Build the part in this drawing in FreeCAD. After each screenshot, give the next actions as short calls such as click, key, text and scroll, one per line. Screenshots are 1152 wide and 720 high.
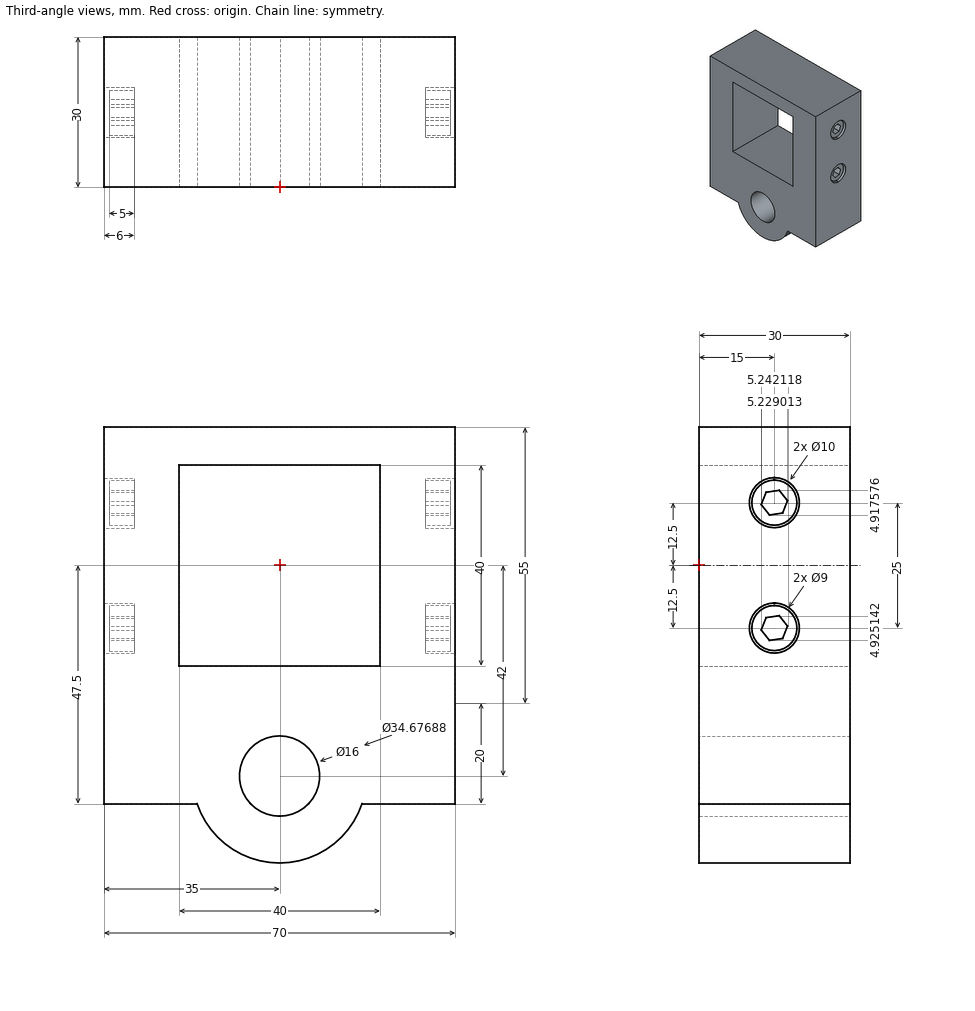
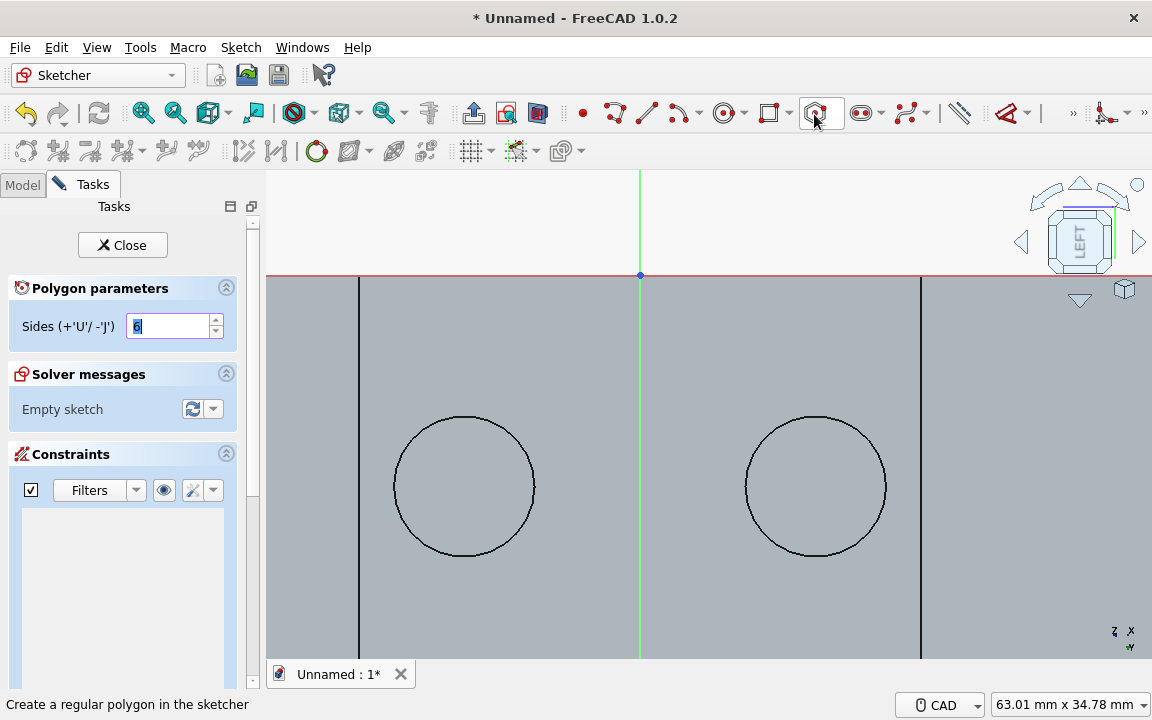
click(816, 487)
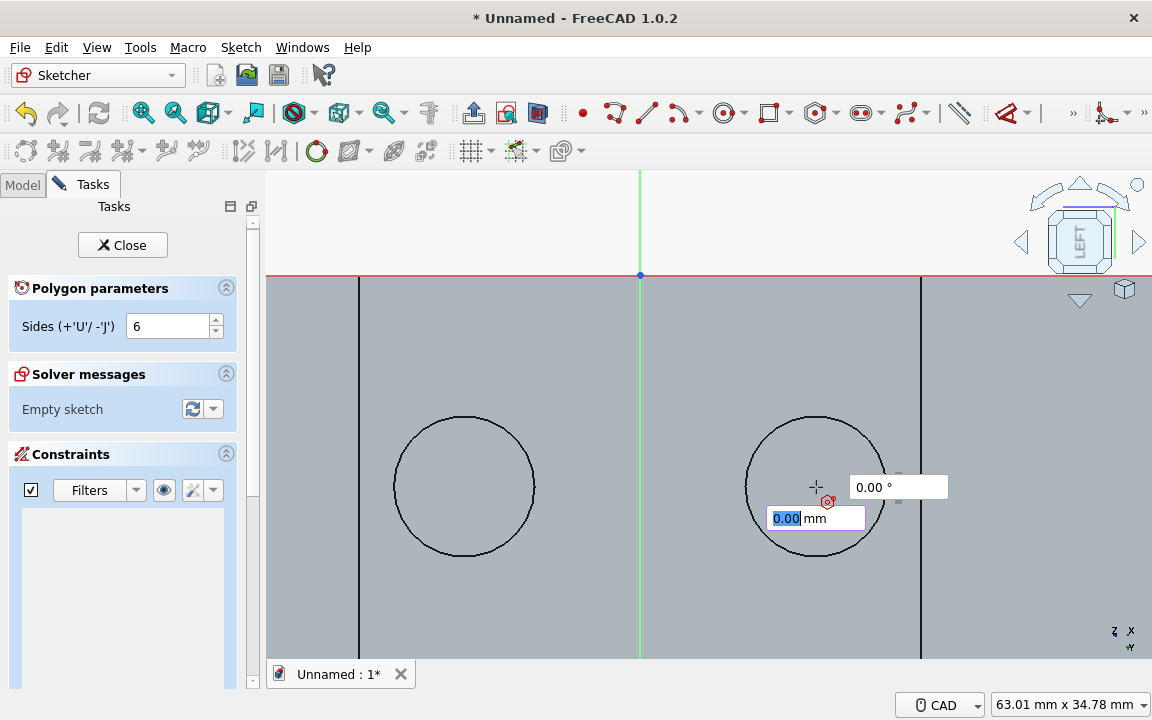
click(845, 510)
right_click(845, 510)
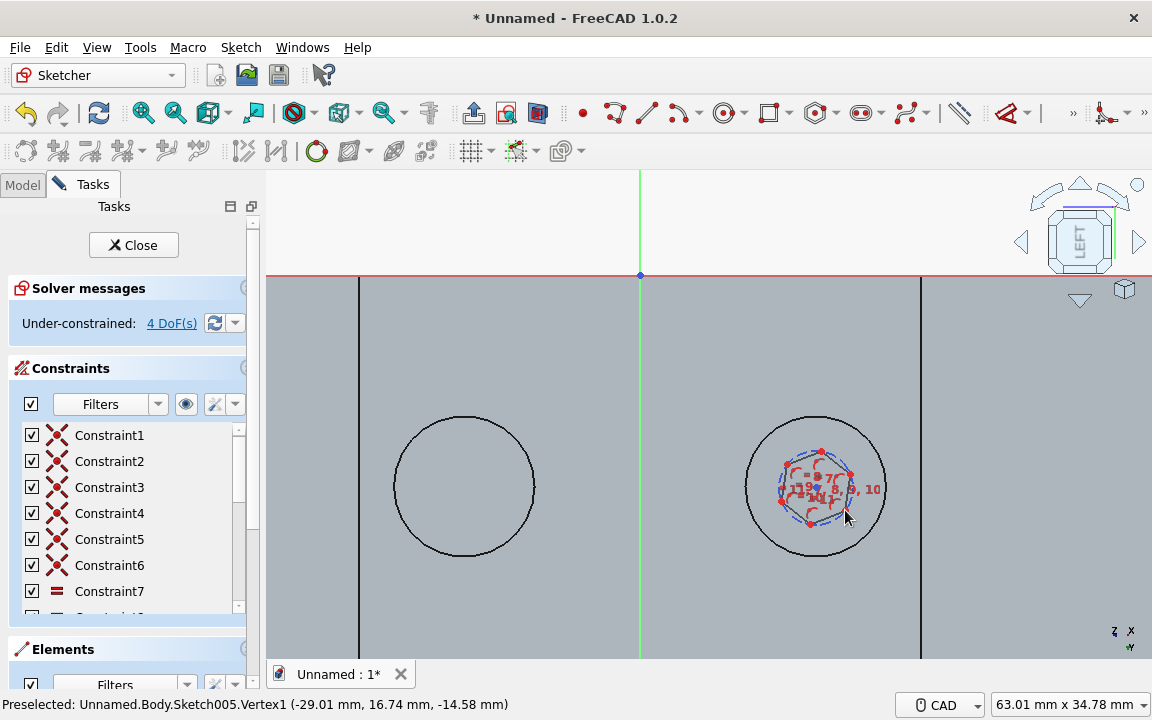
click(816, 114)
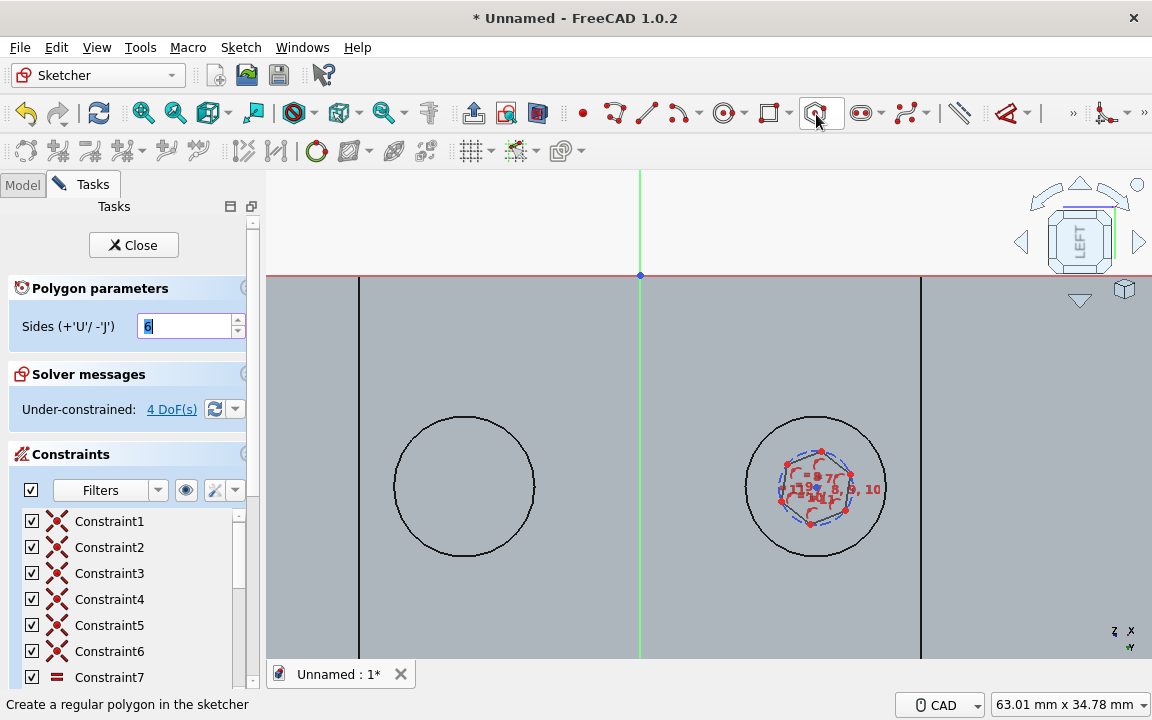
click(464, 487)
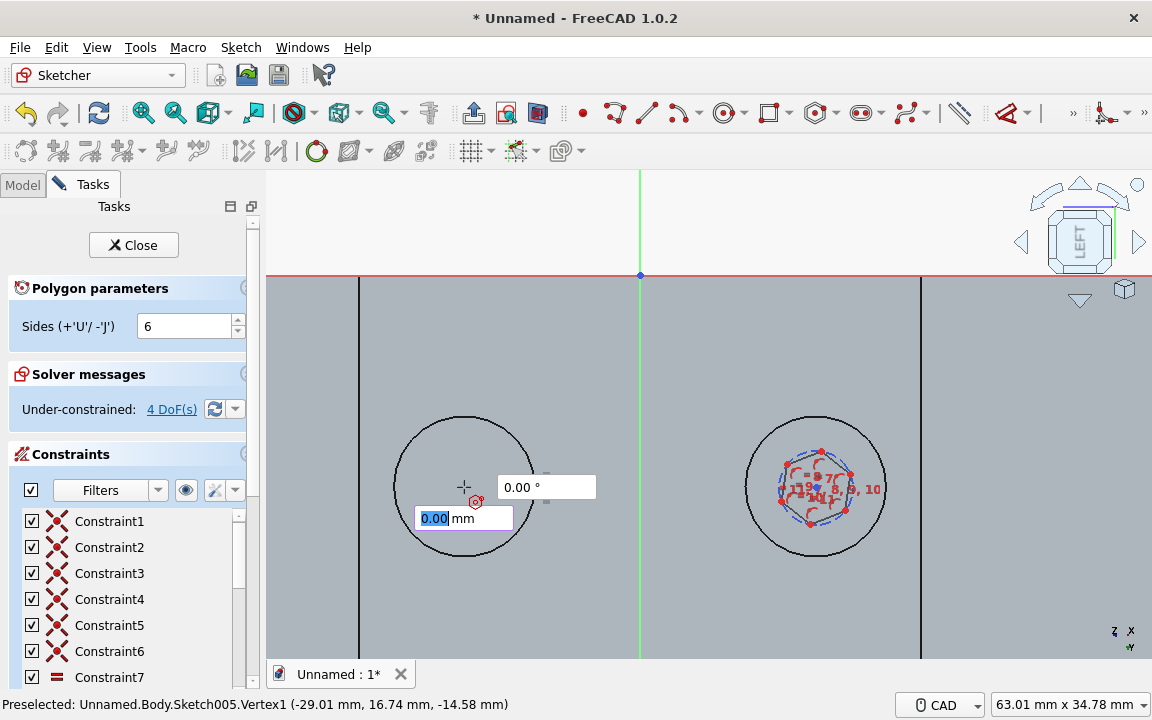
click(430, 500)
right_click(430, 500)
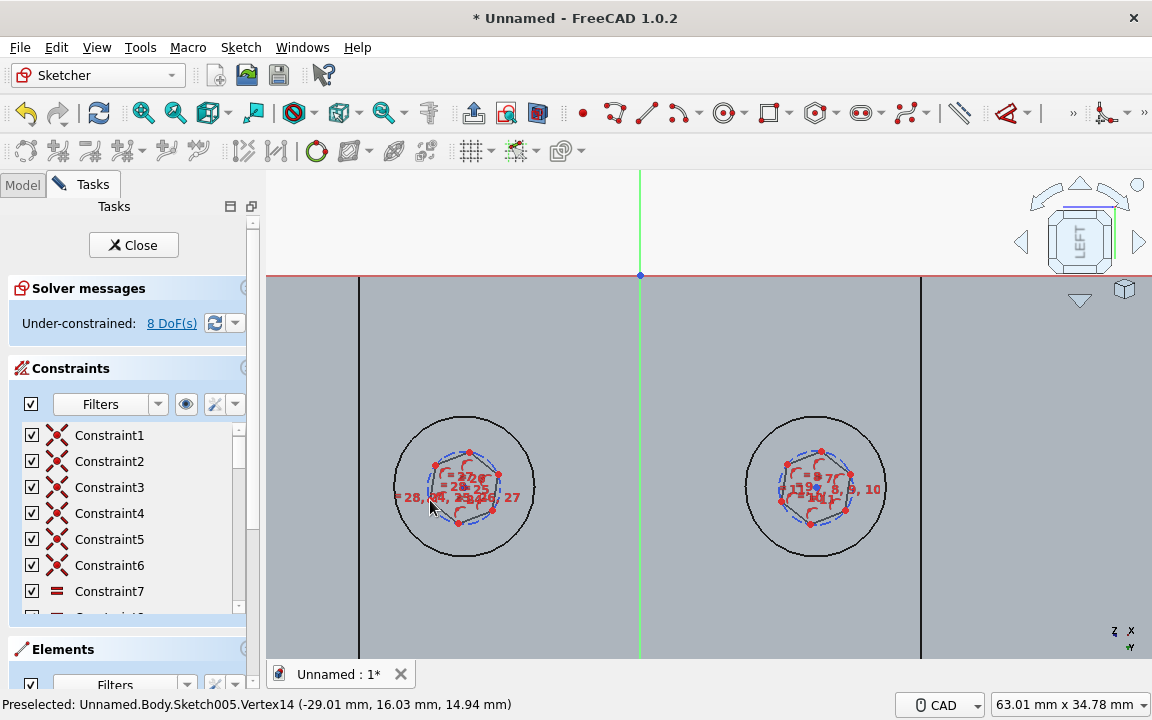
click(724, 114)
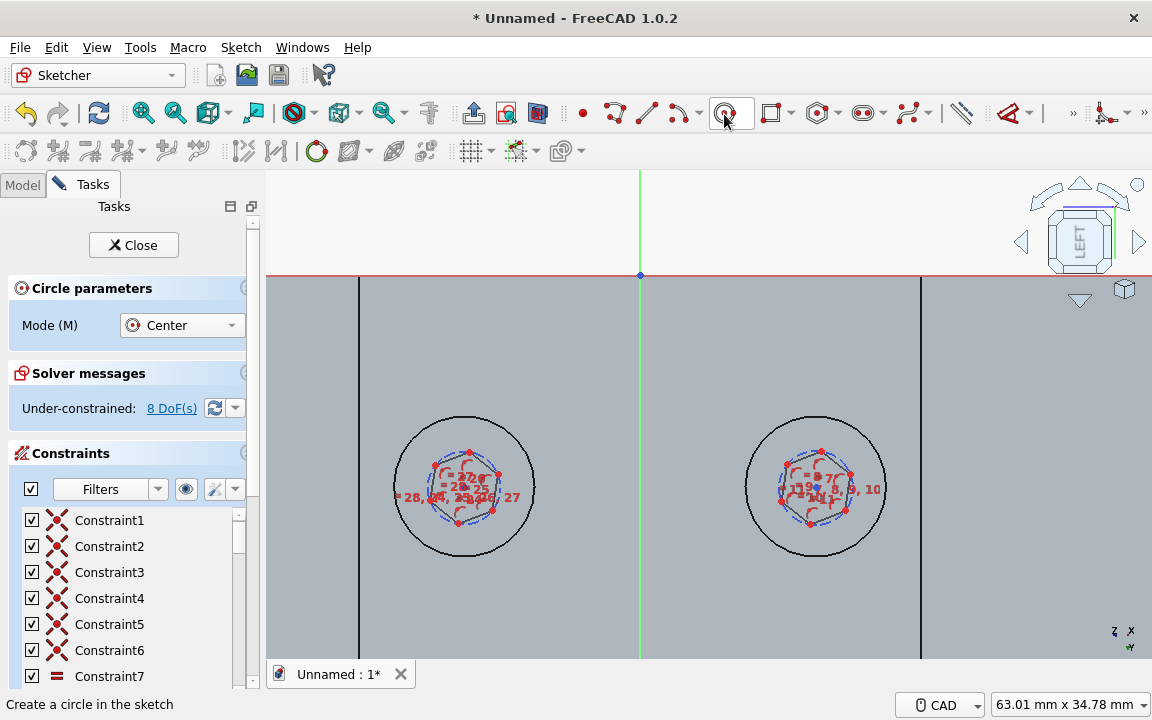
click(816, 488)
move(861, 442)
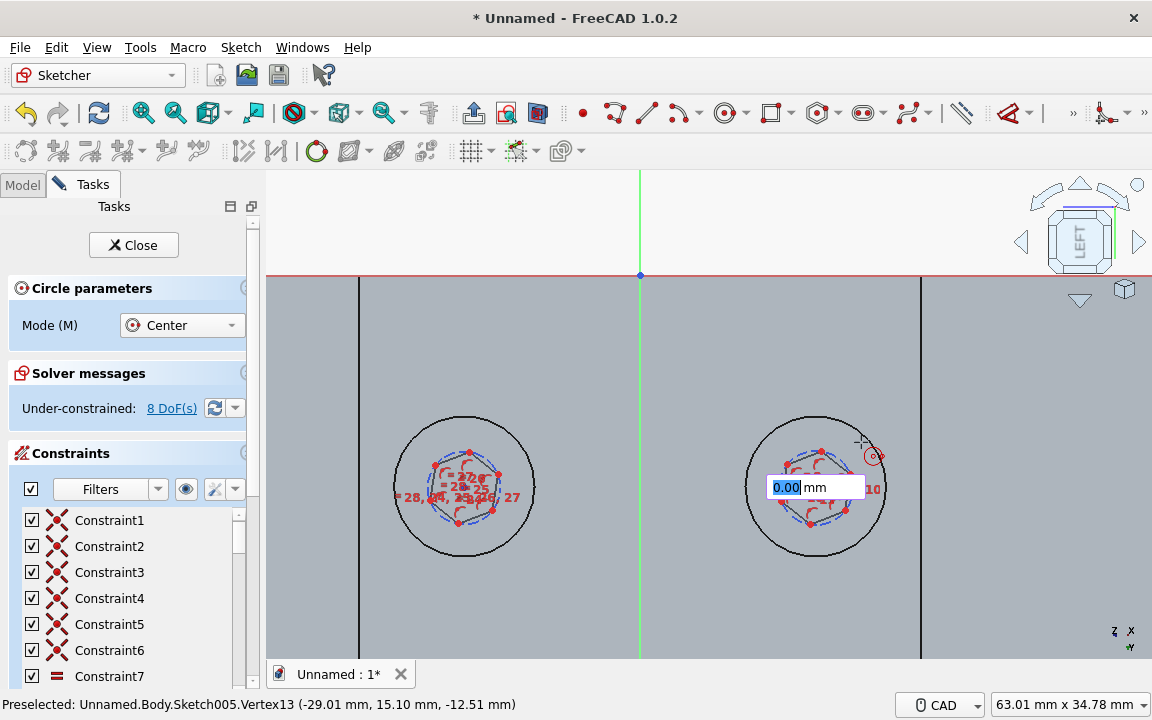
text(9)
key(Return)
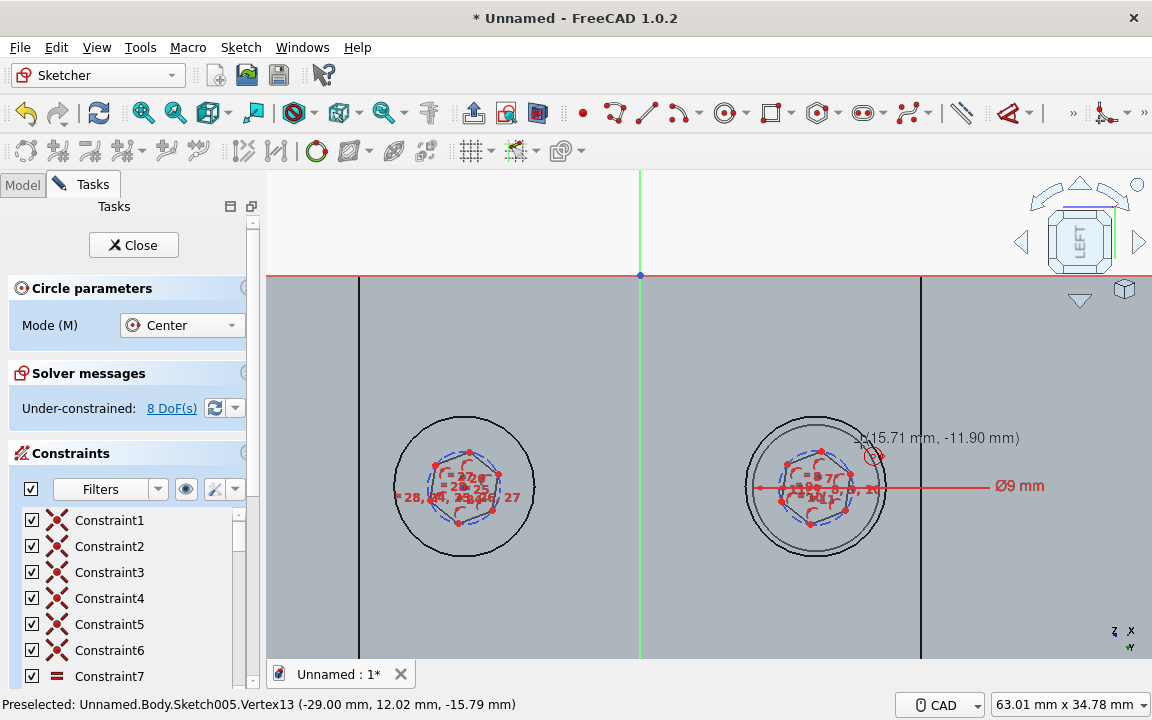
click(464, 488)
move(509, 442)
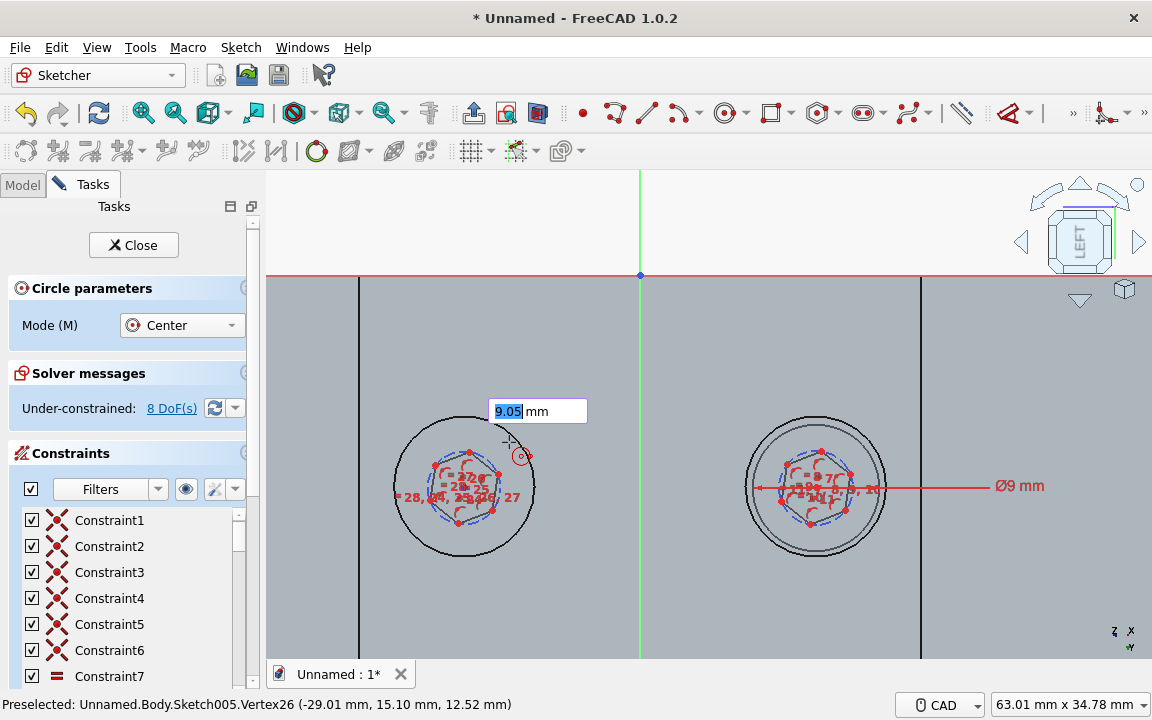
text(9)
key(Return)
key(Escape)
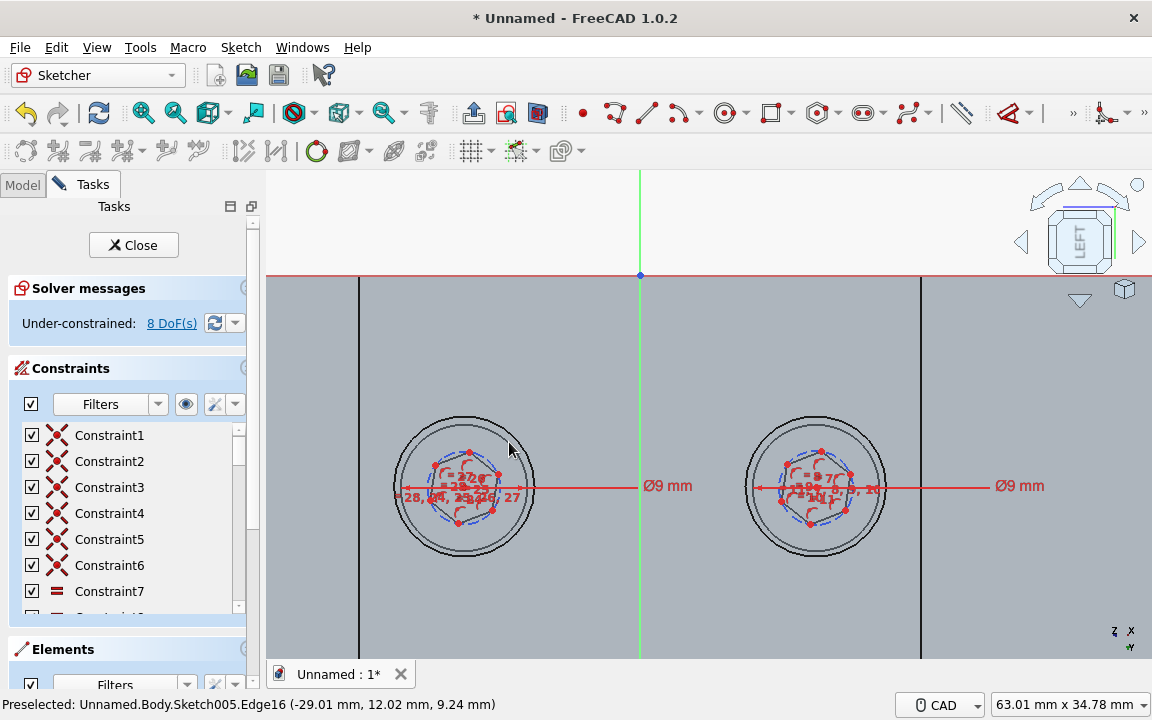
click(816, 488)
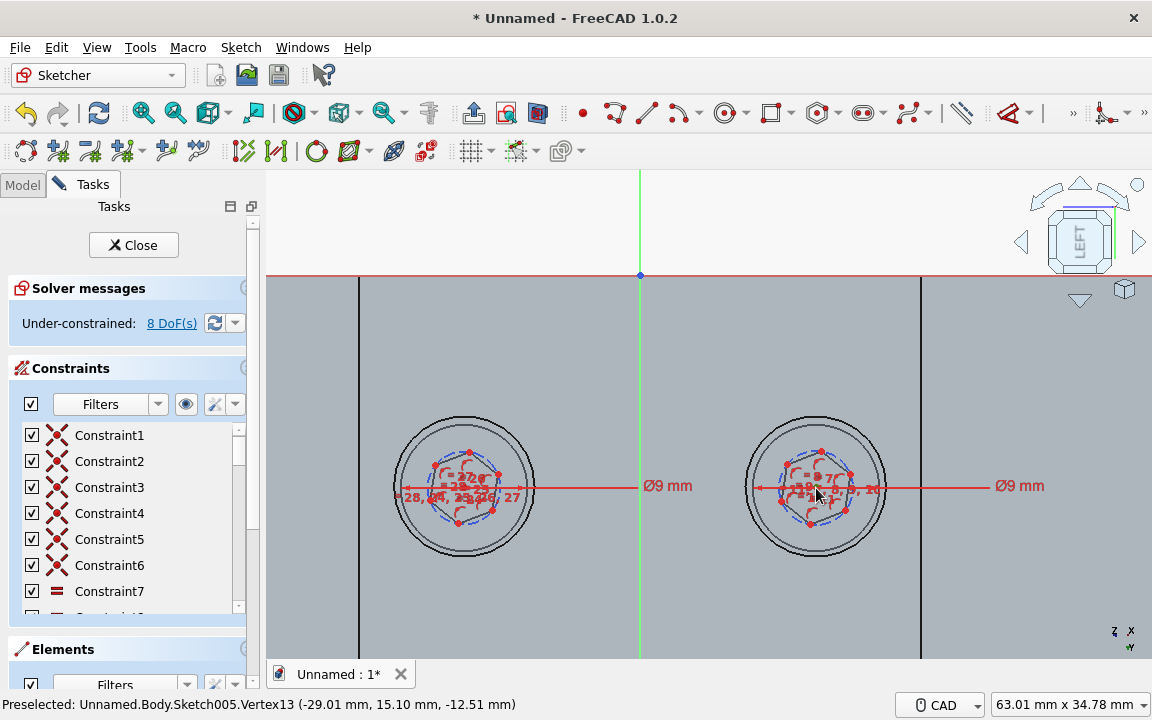
scroll(464, 488, up, 4)